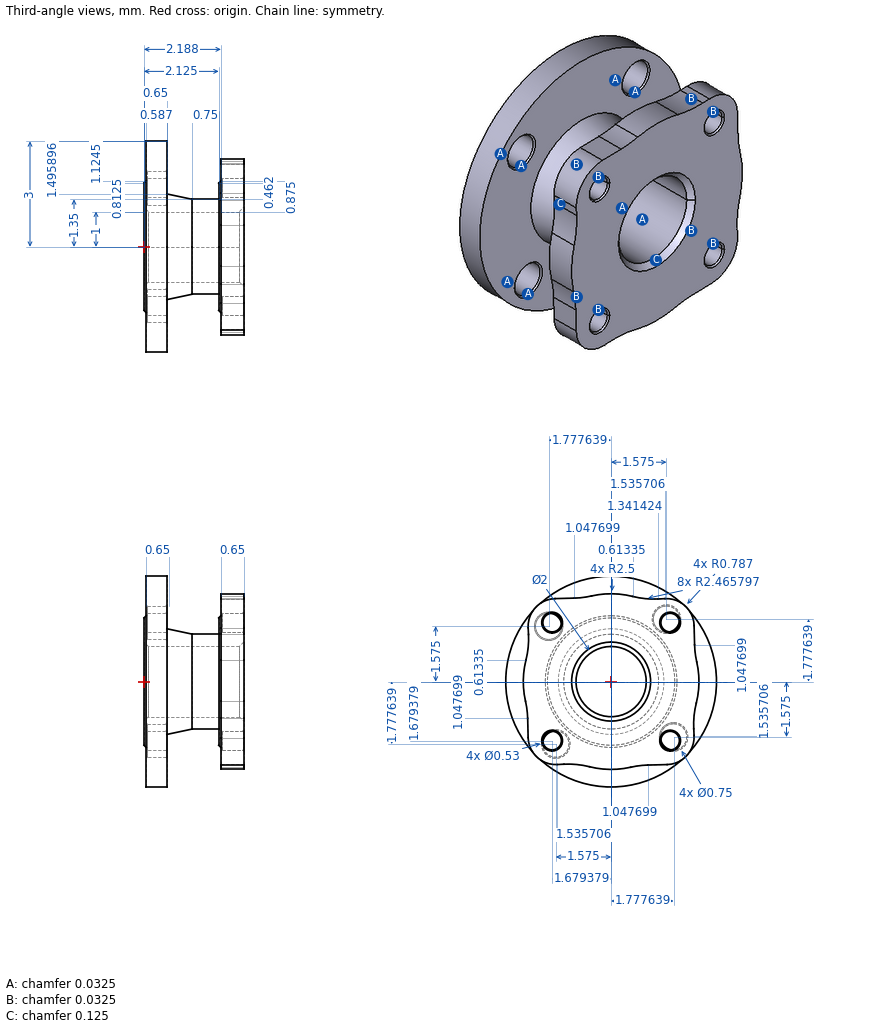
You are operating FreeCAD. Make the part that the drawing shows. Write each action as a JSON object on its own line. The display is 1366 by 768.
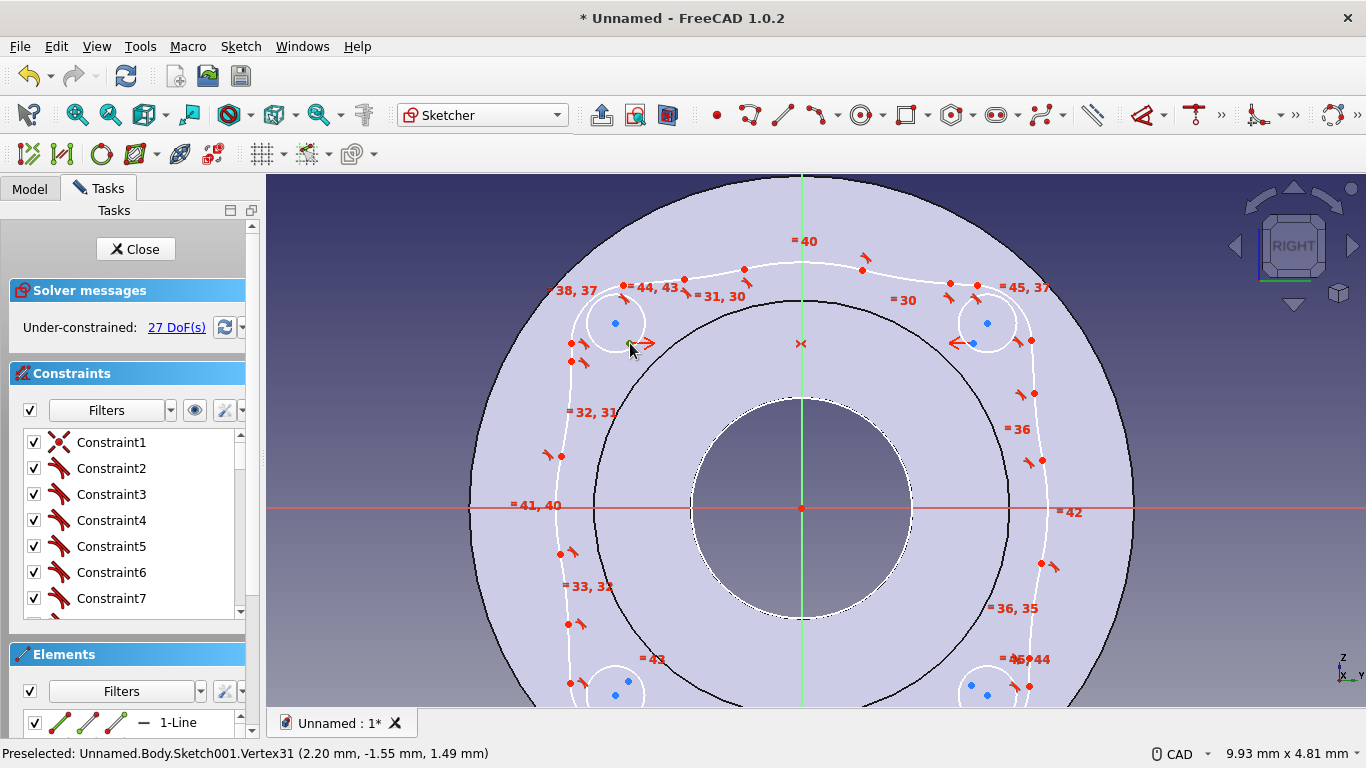
{"action": "scroll", "coordinate": [637, 303], "scroll_direction": "down", "scroll_amount": 2}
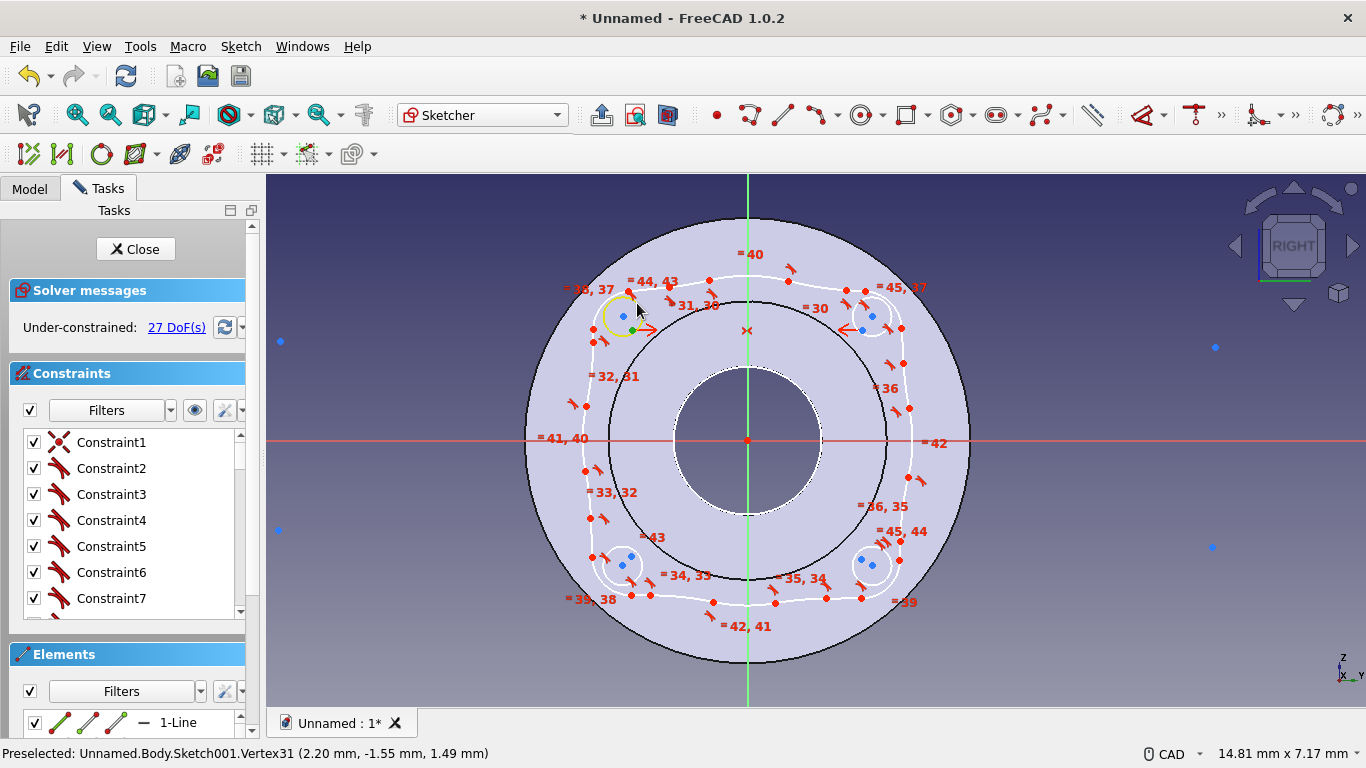
{"action": "left_click", "coordinate": [631, 556]}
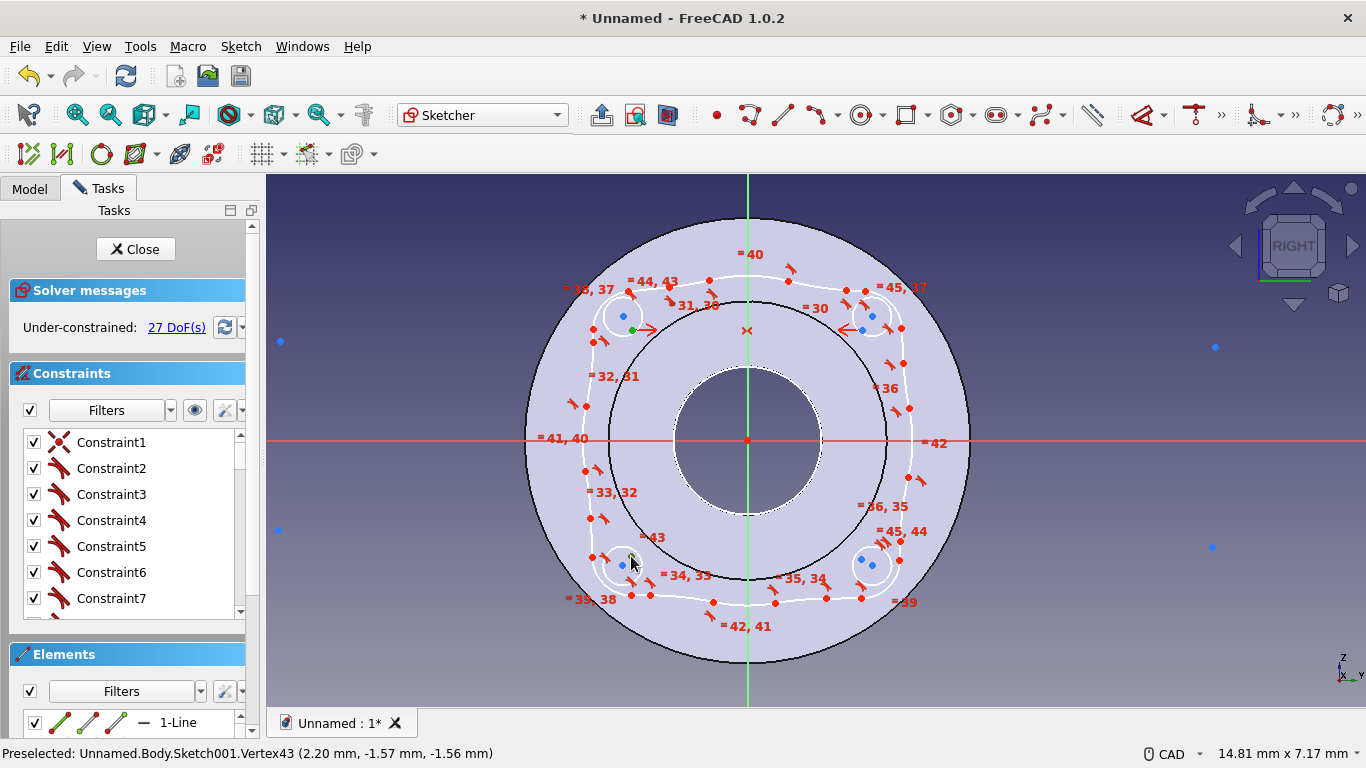
{"action": "left_click", "coordinate": [359, 441]}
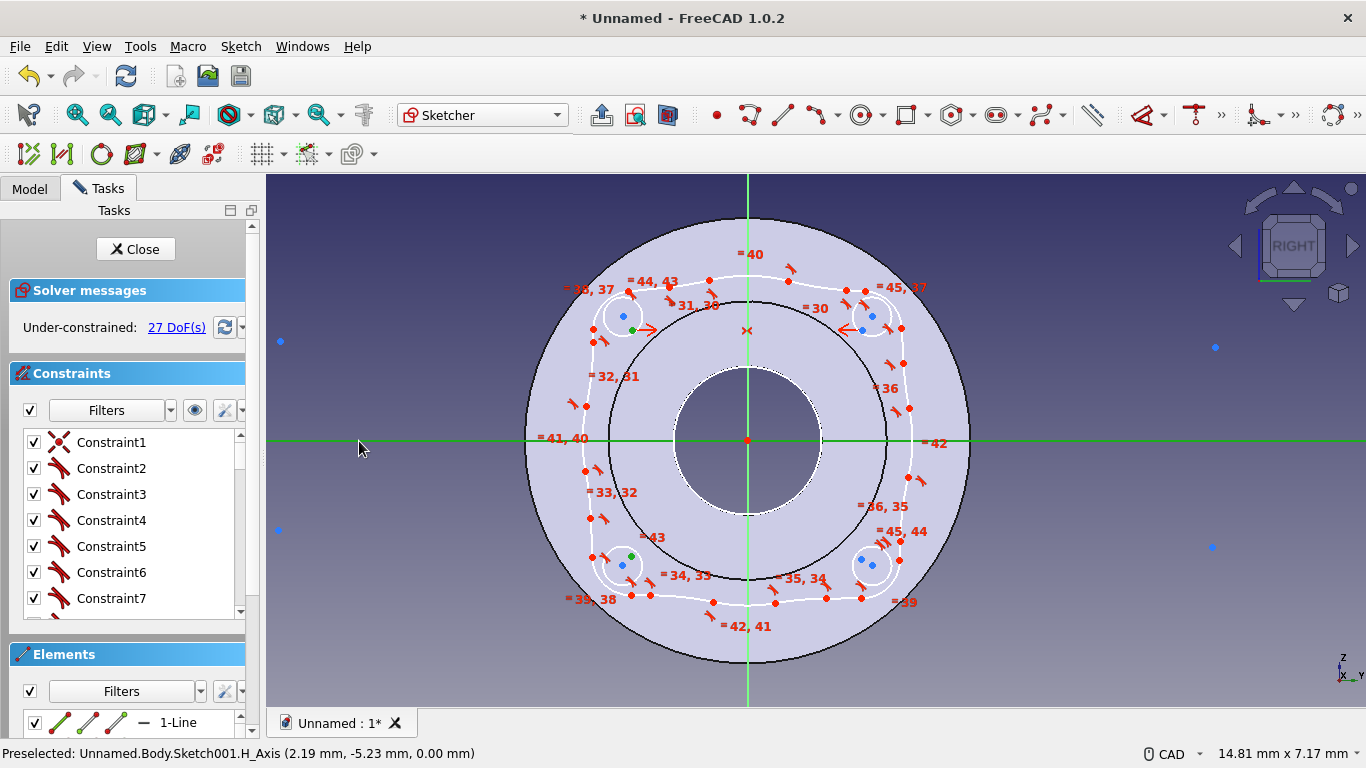
{"action": "key", "text": "s"}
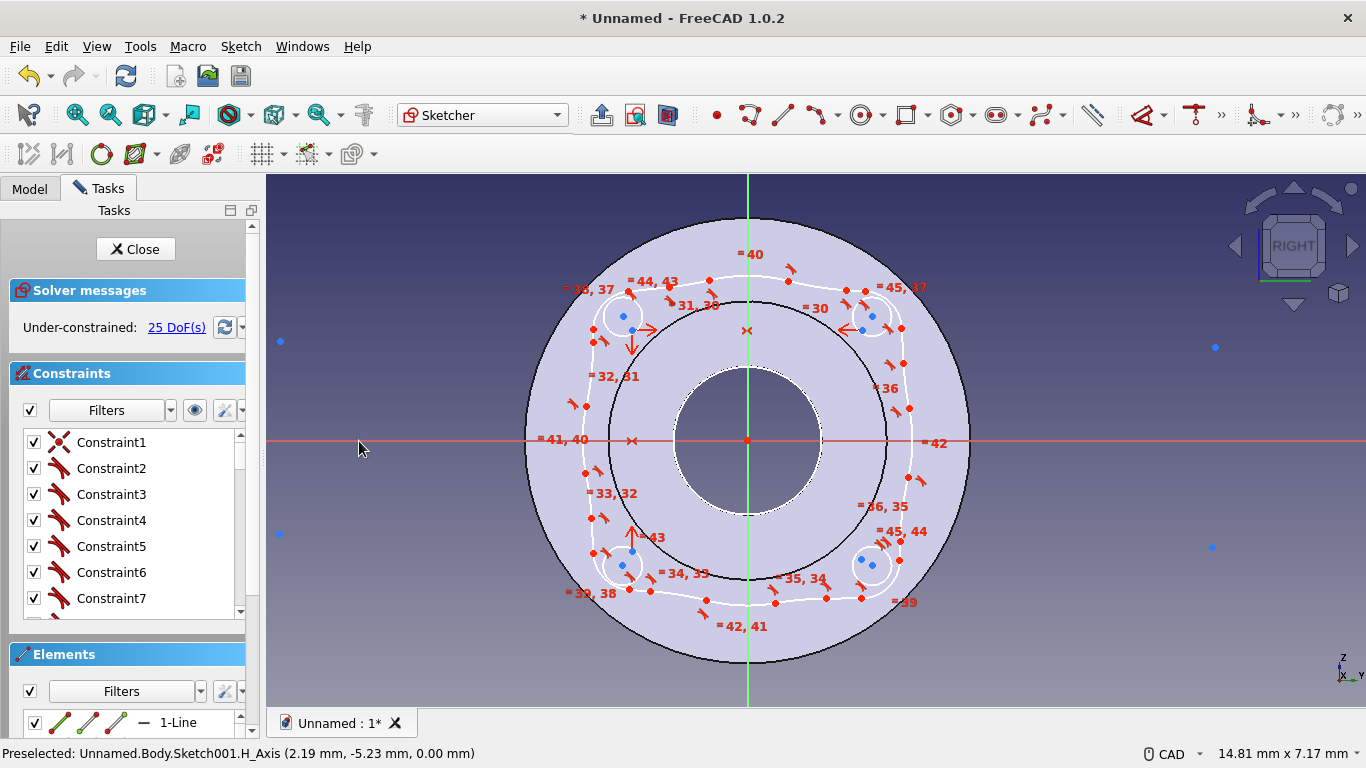
{"action": "left_click", "coordinate": [863, 330]}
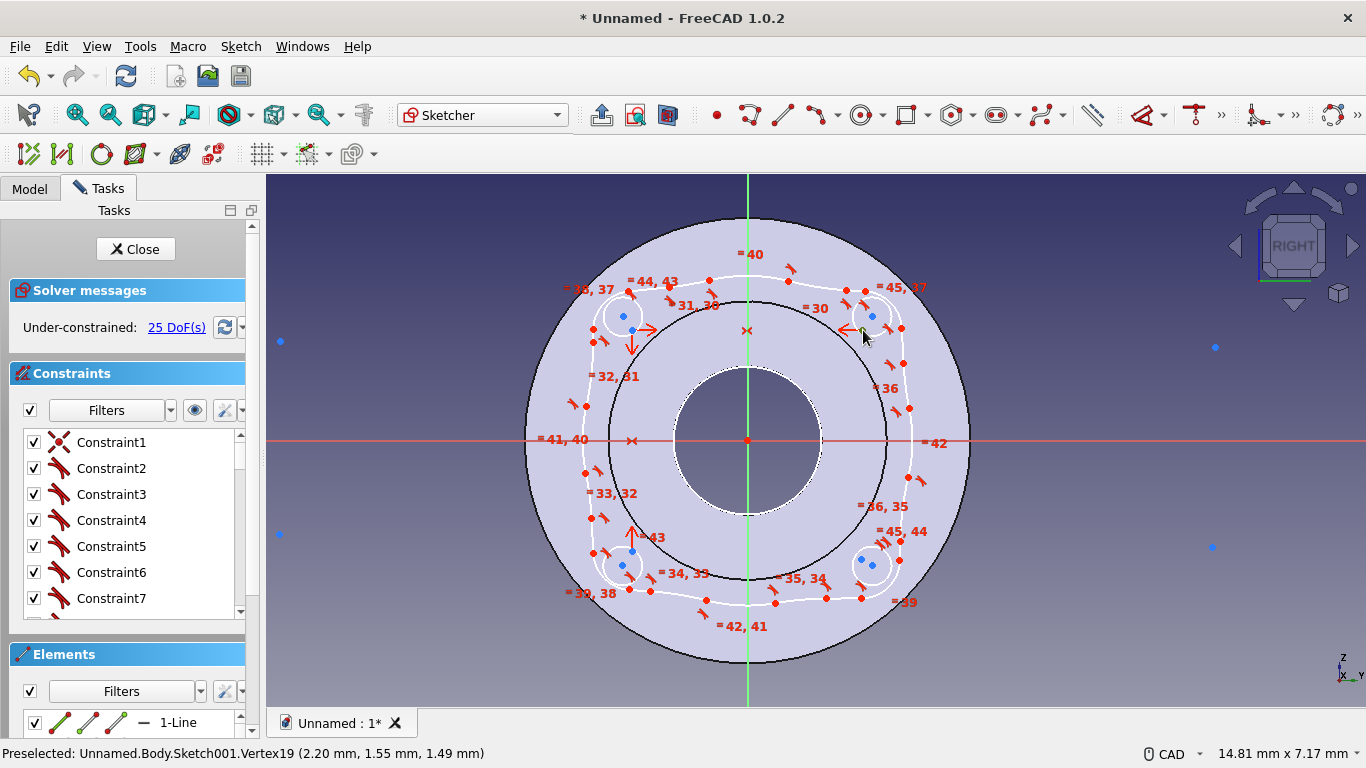
{"action": "left_click", "coordinate": [861, 560]}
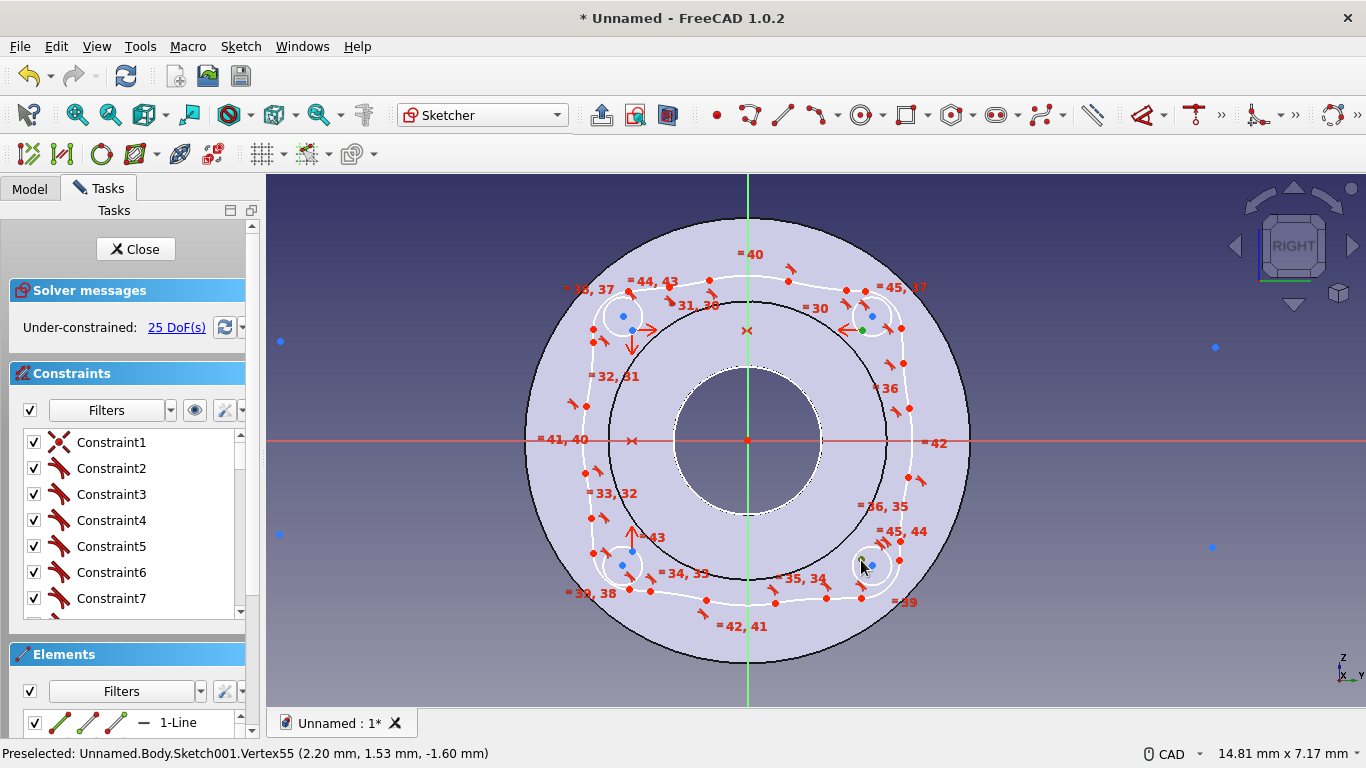
{"action": "left_click", "coordinate": [359, 441]}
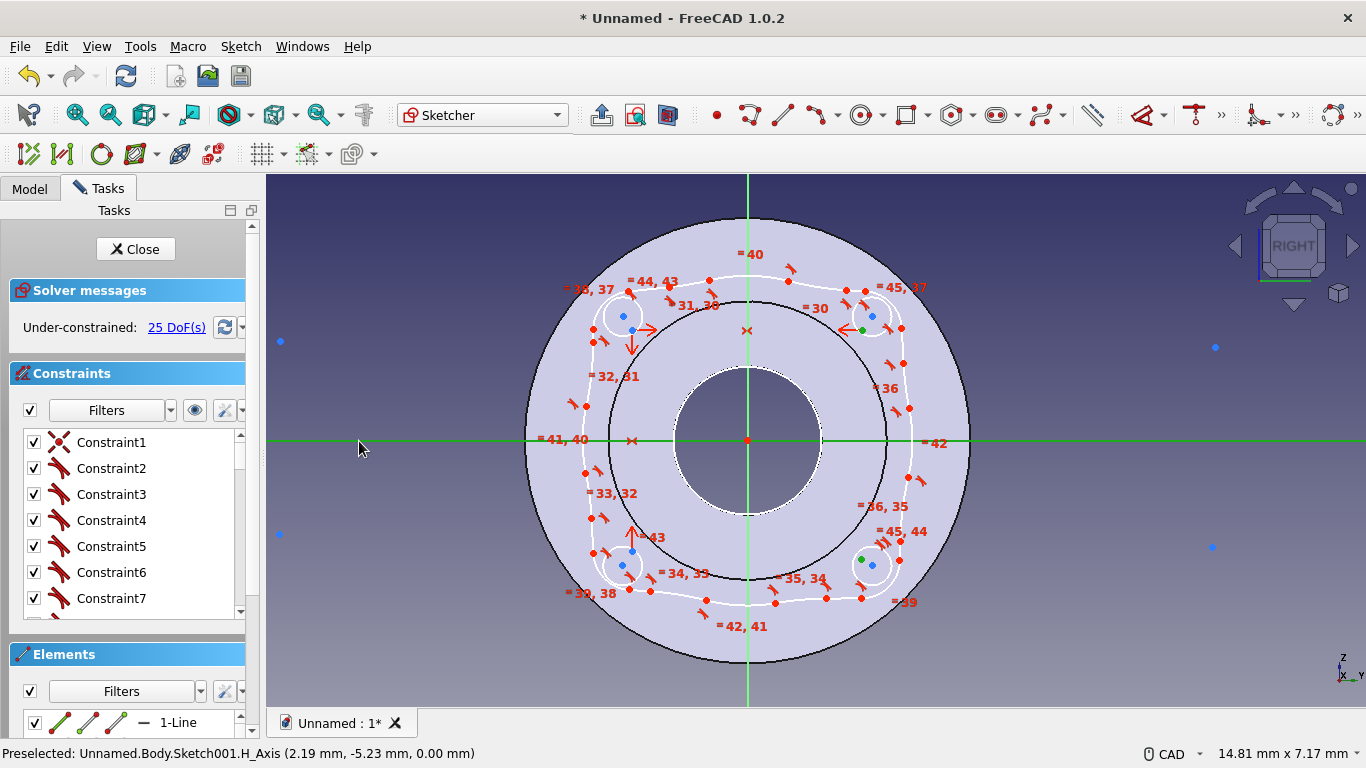
{"action": "key", "text": "s"}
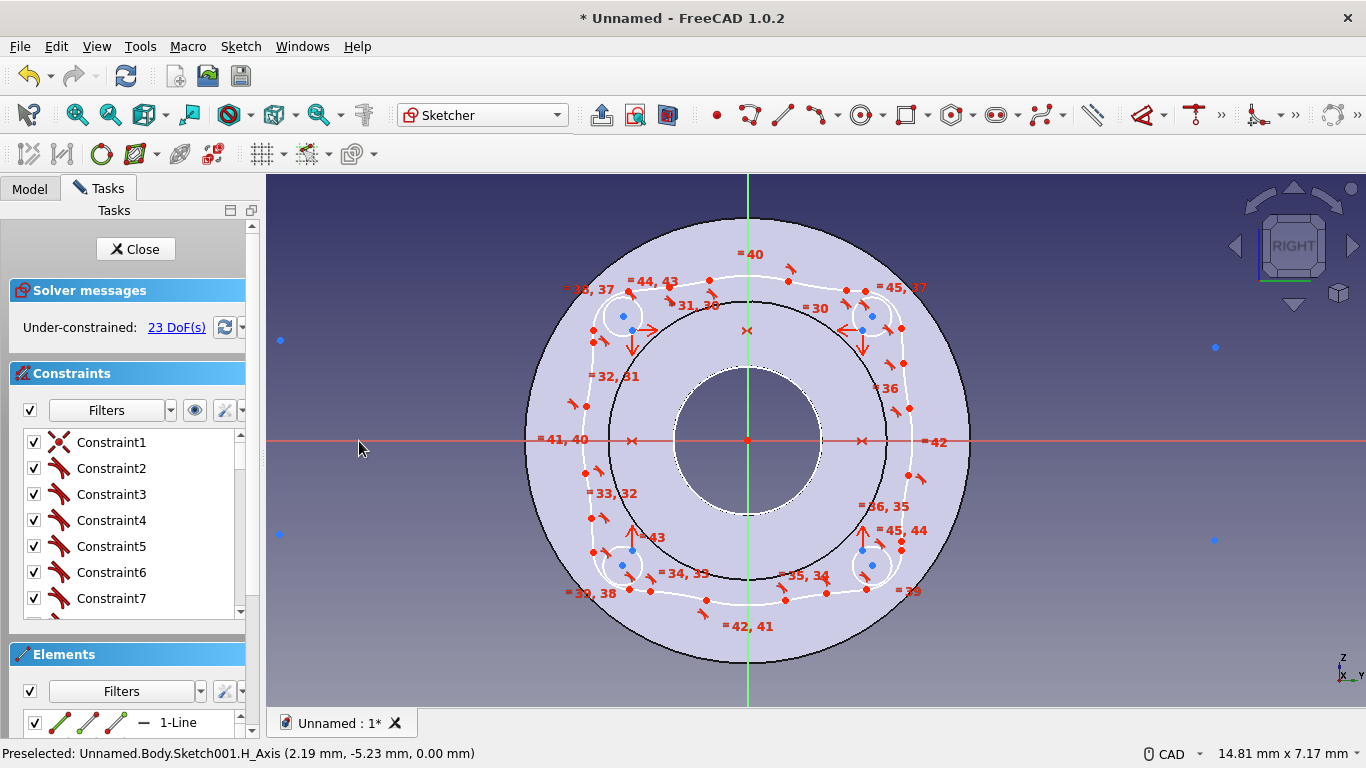
{"action": "left_click", "coordinate": [623, 566]}